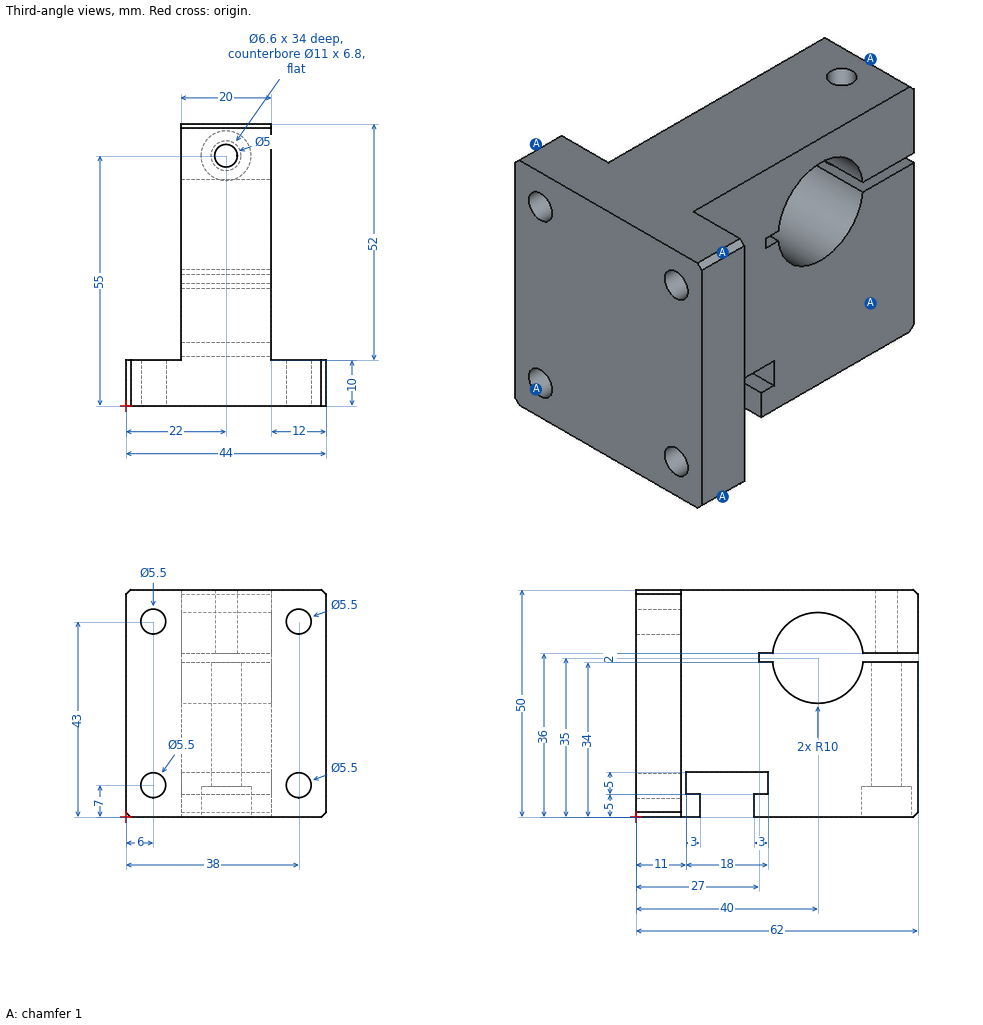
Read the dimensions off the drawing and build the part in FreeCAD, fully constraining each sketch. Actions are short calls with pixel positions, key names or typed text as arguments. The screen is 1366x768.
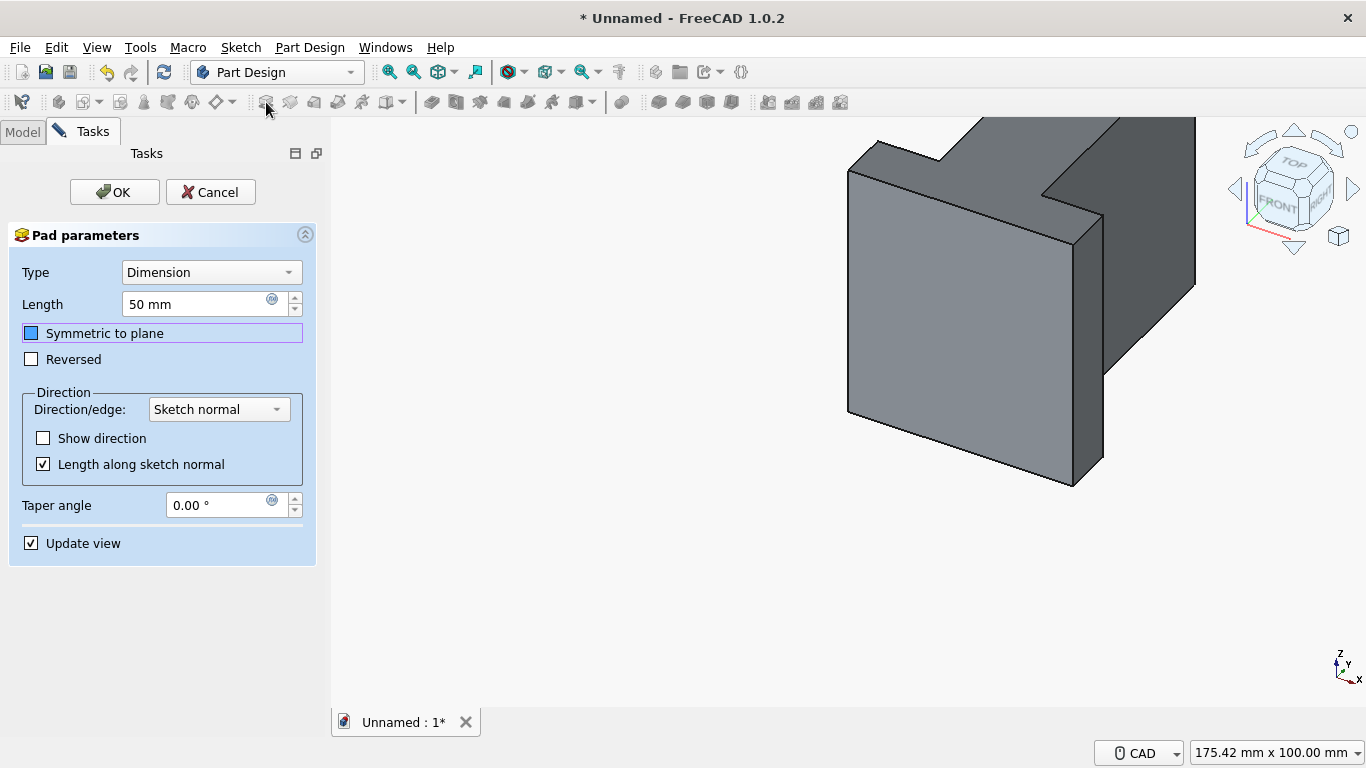
click(115, 192)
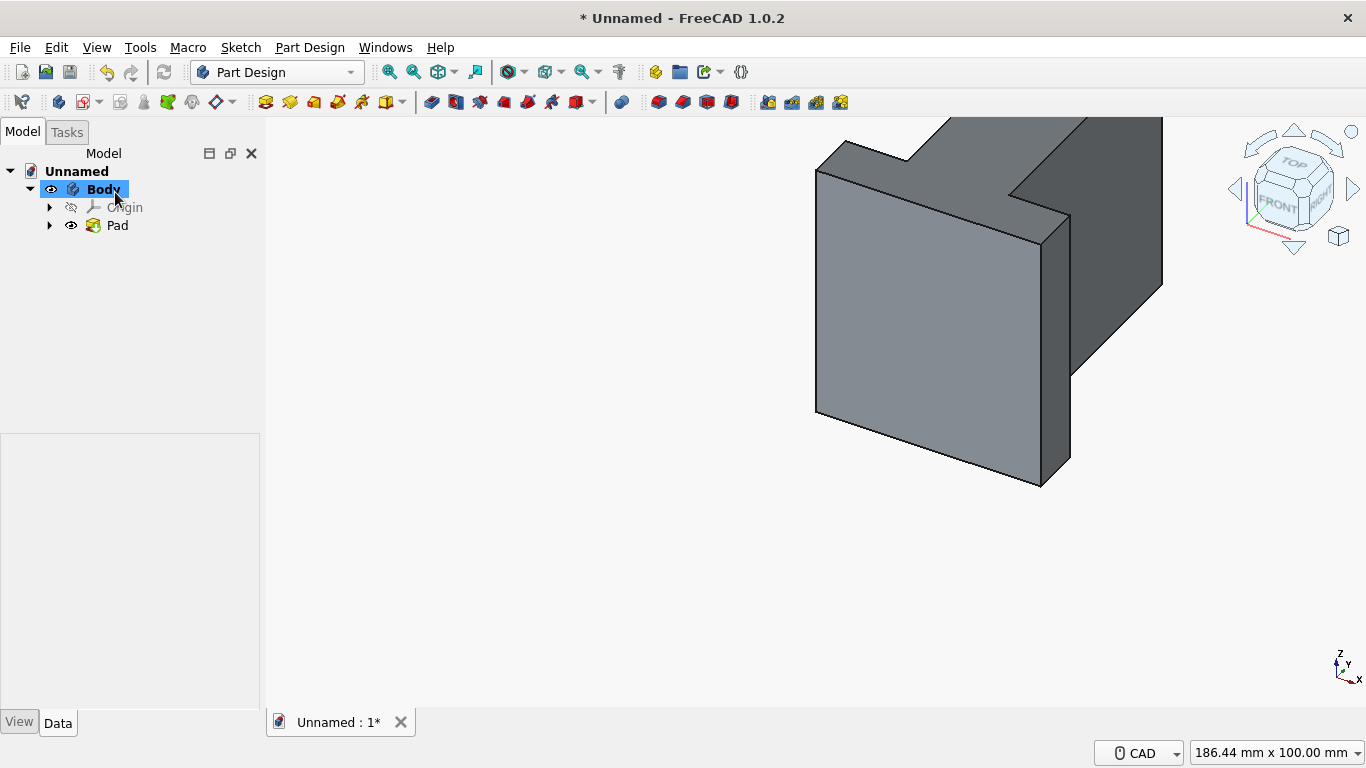
click(390, 72)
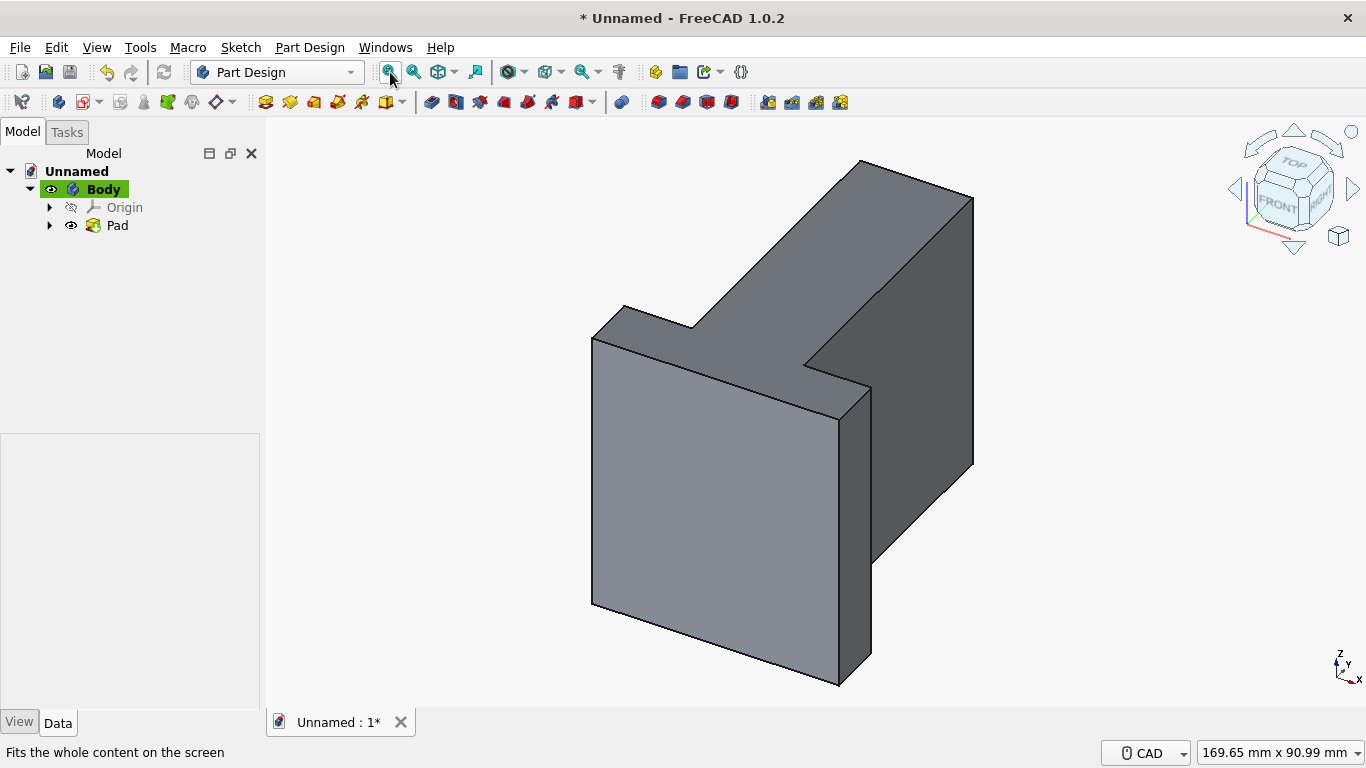
click(715, 511)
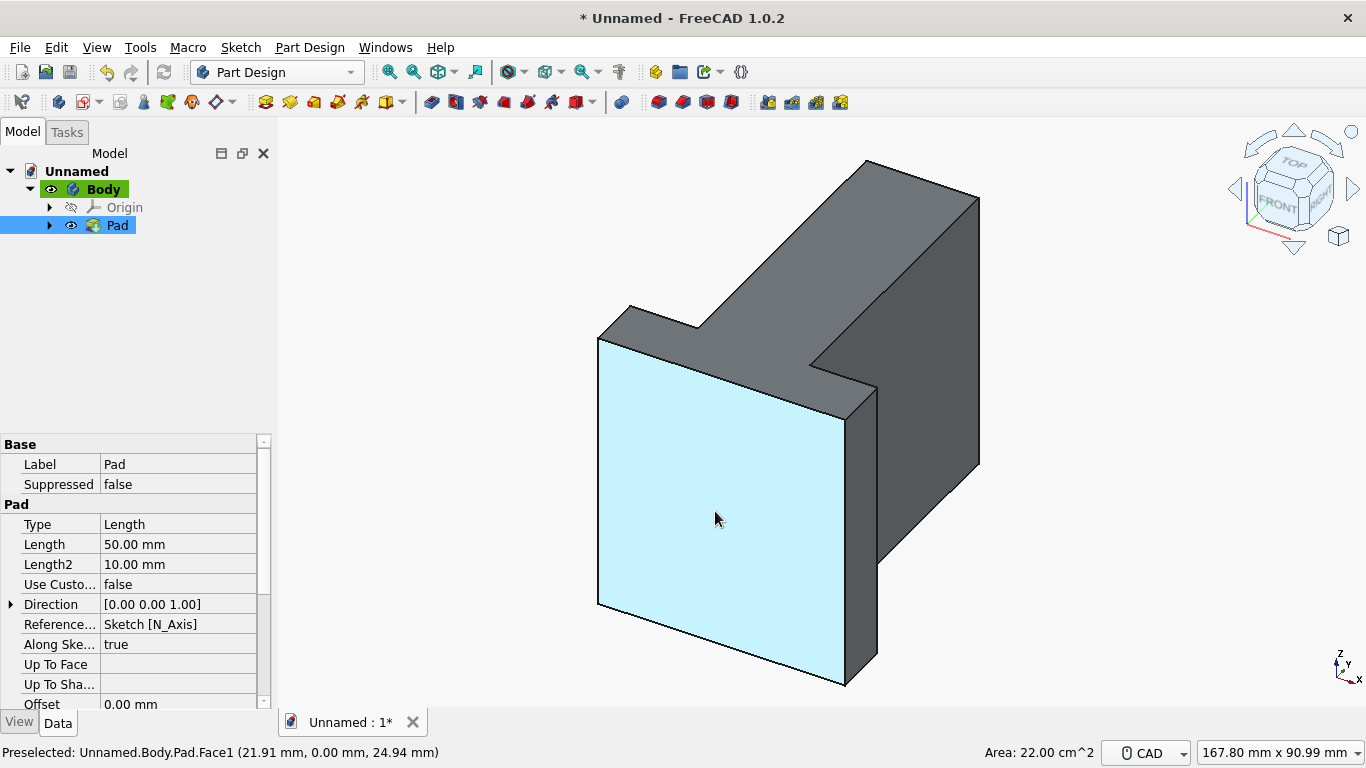
click(84, 102)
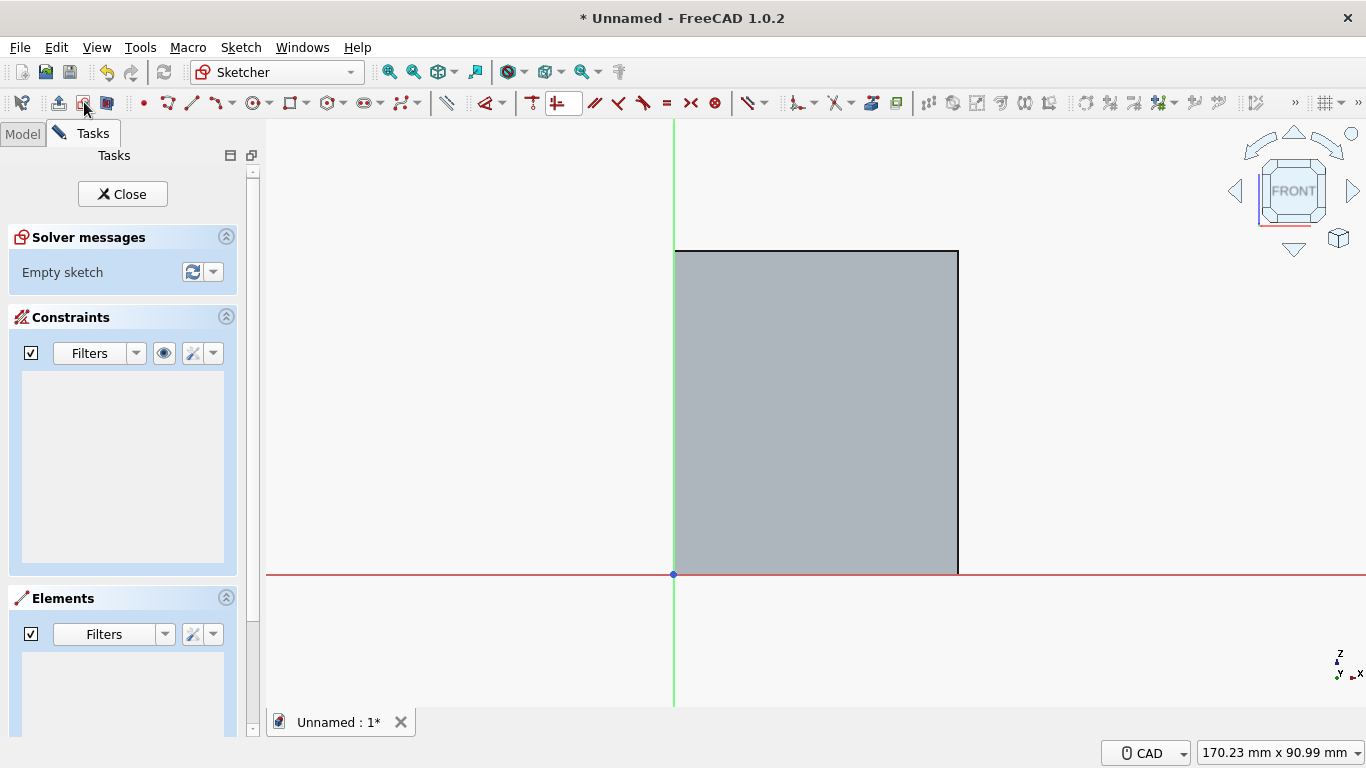
scroll(709, 285, up, 12)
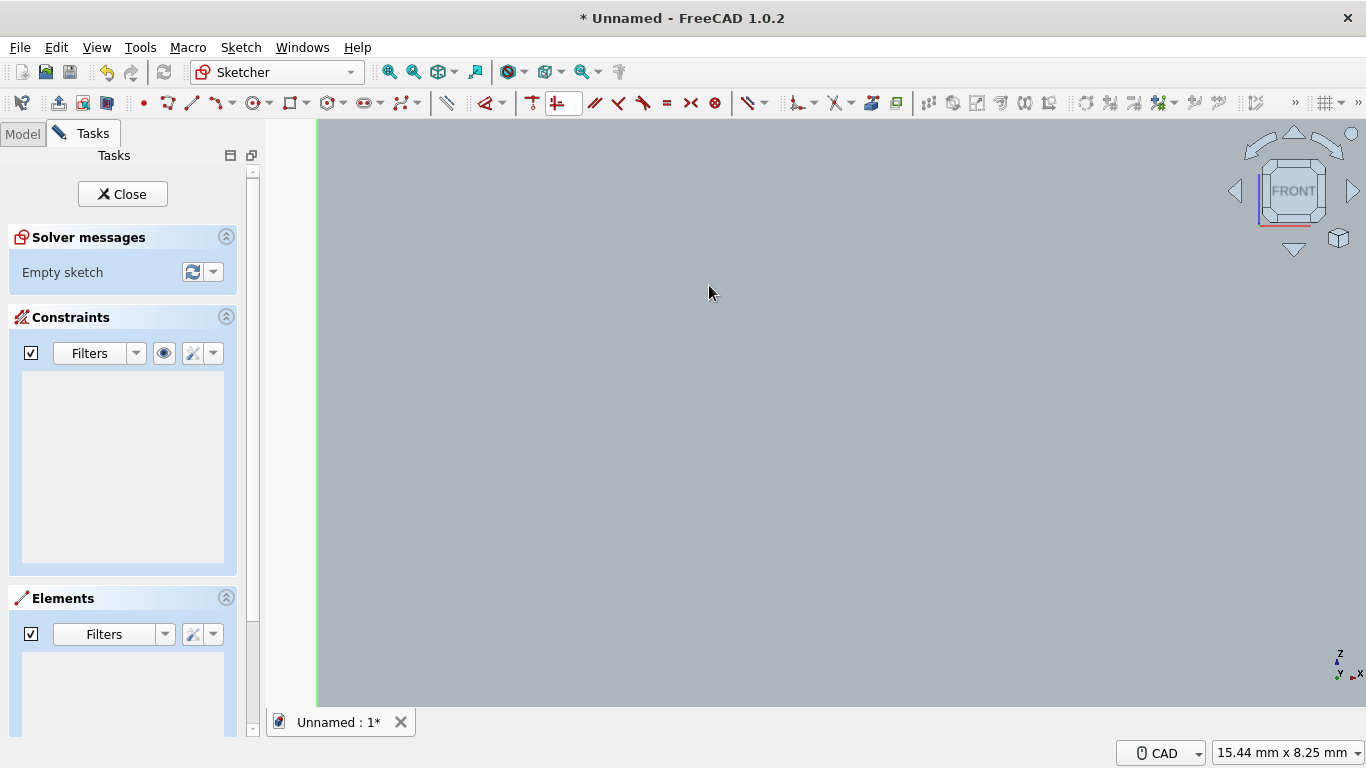
click(254, 104)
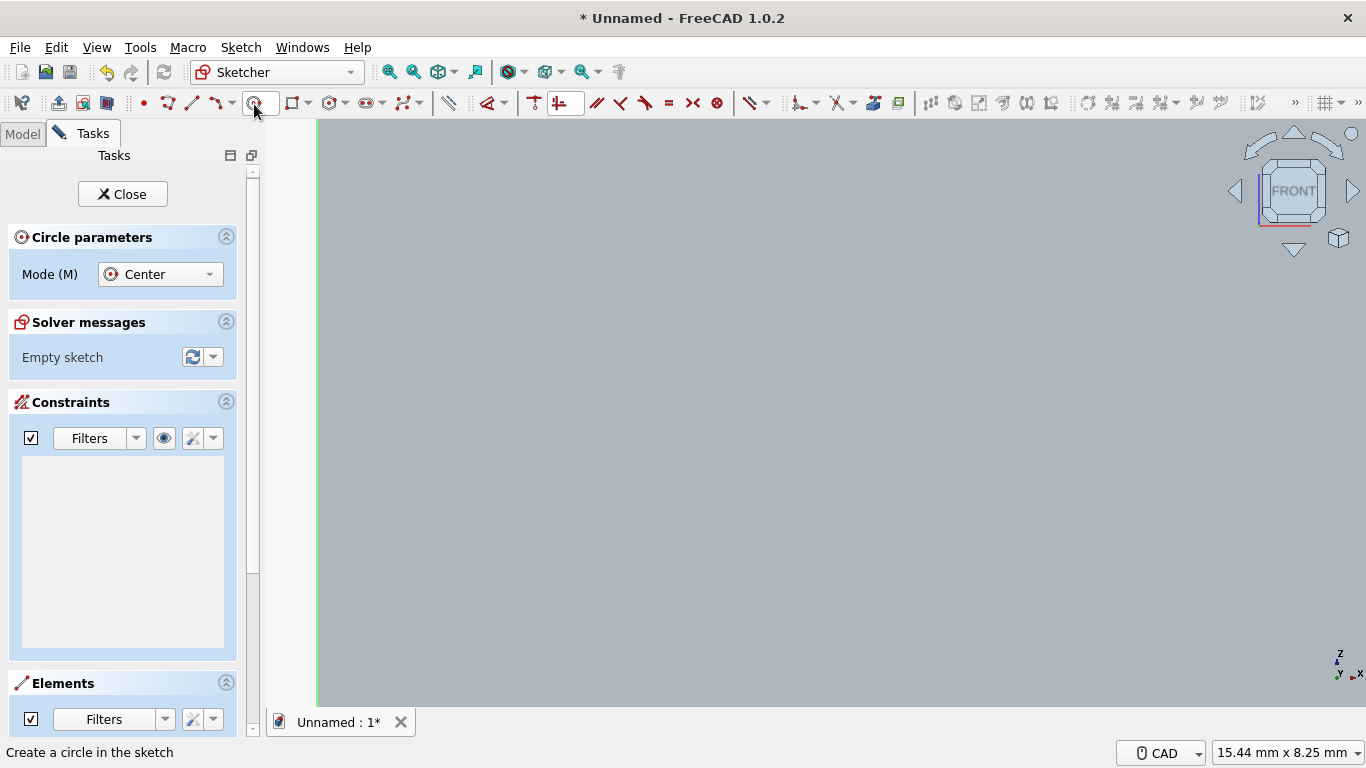
click(745, 411)
move(883, 272)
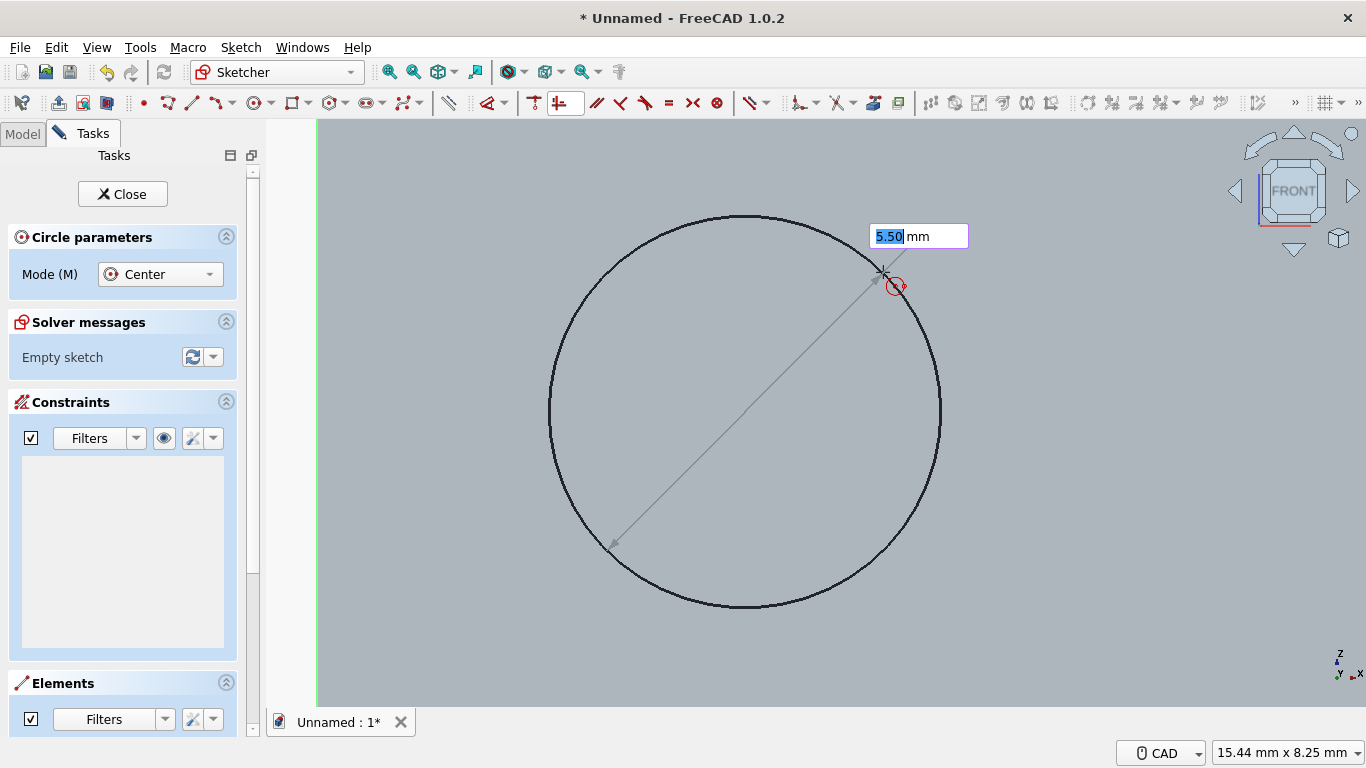
text(5.5)
key(Return)
key(Escape)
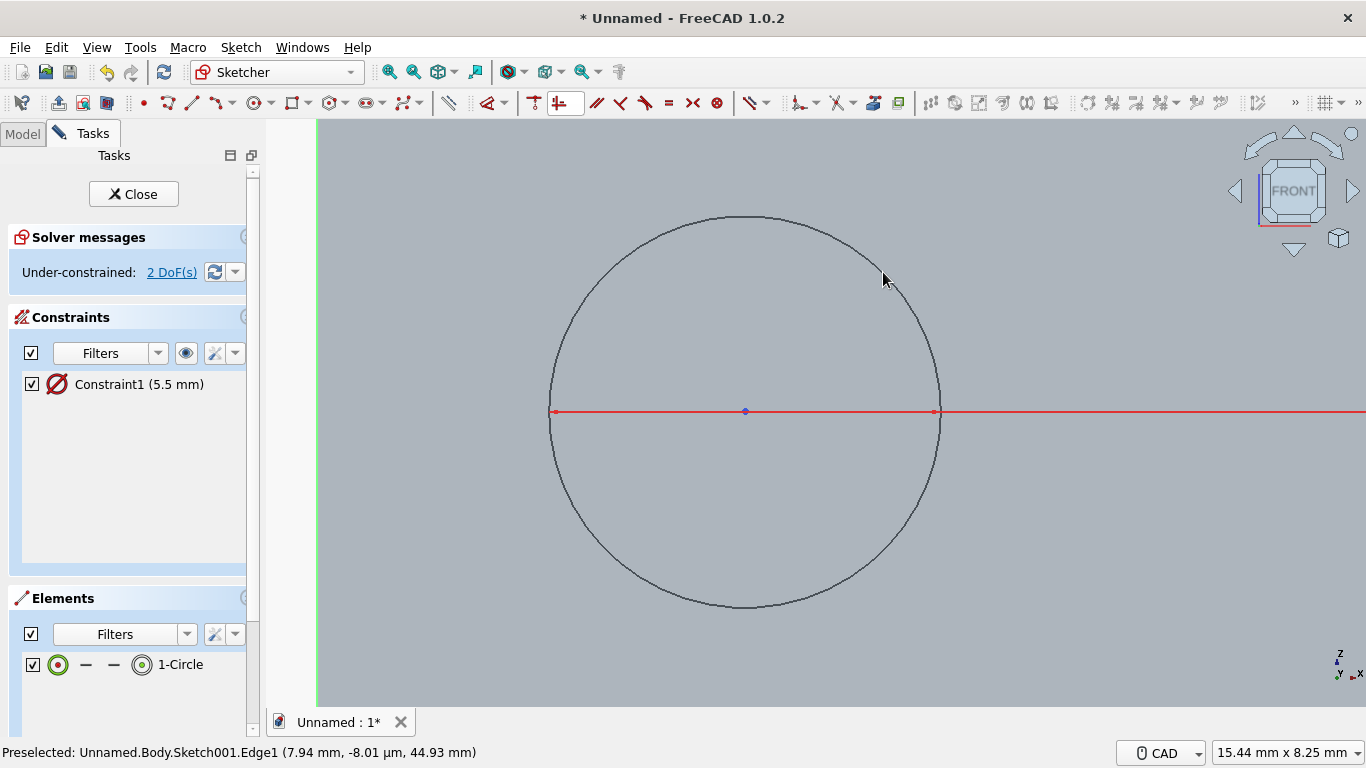
click(488, 104)